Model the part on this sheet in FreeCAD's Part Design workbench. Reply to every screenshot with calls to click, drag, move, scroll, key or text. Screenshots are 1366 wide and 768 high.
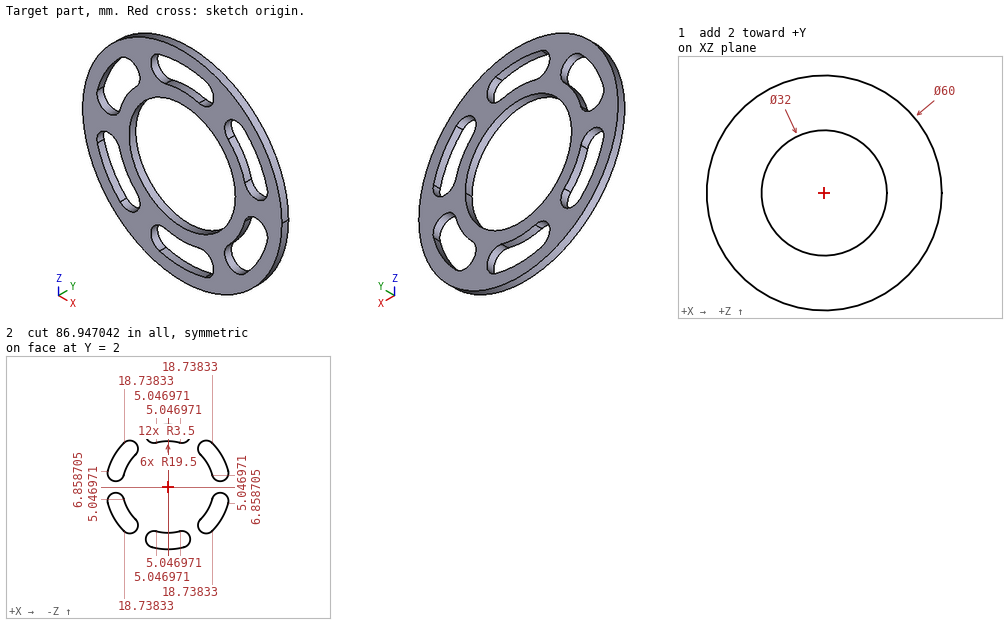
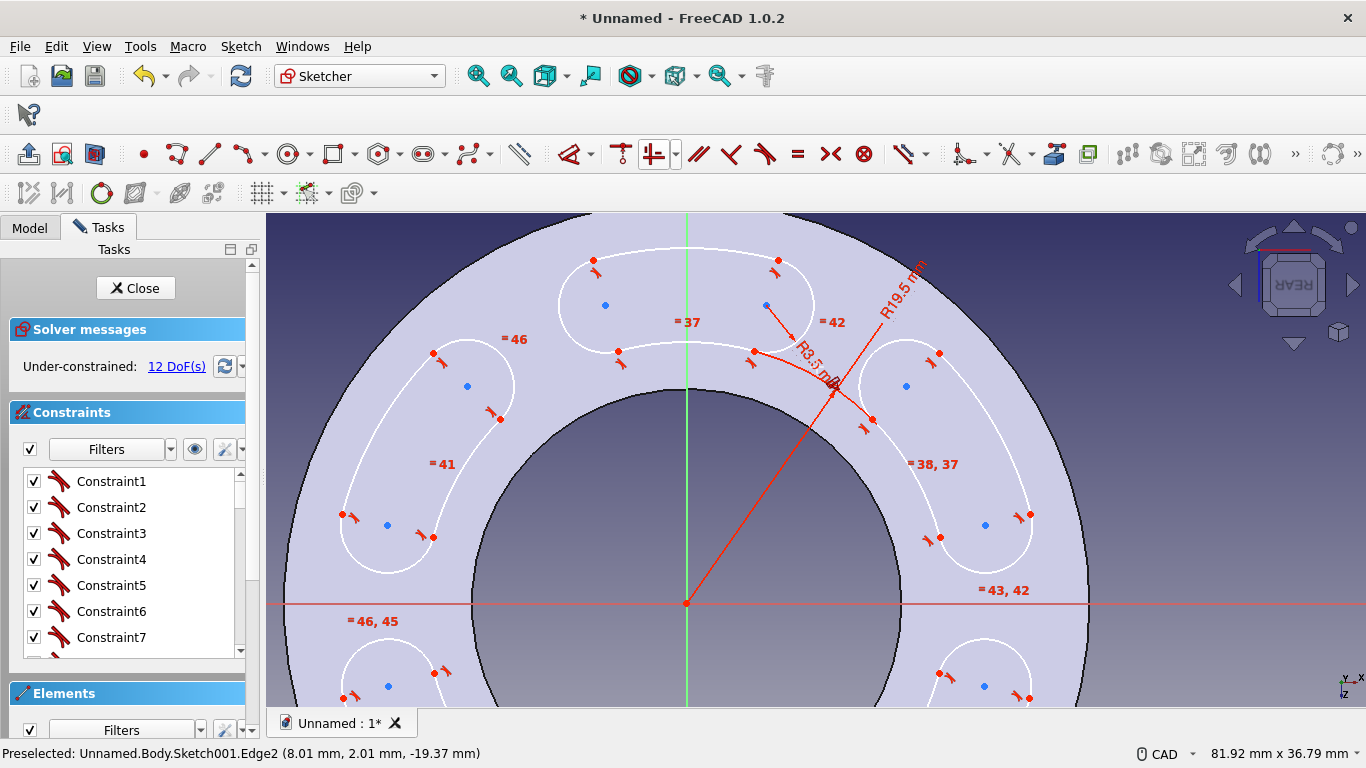
click(755, 351)
click(721, 317)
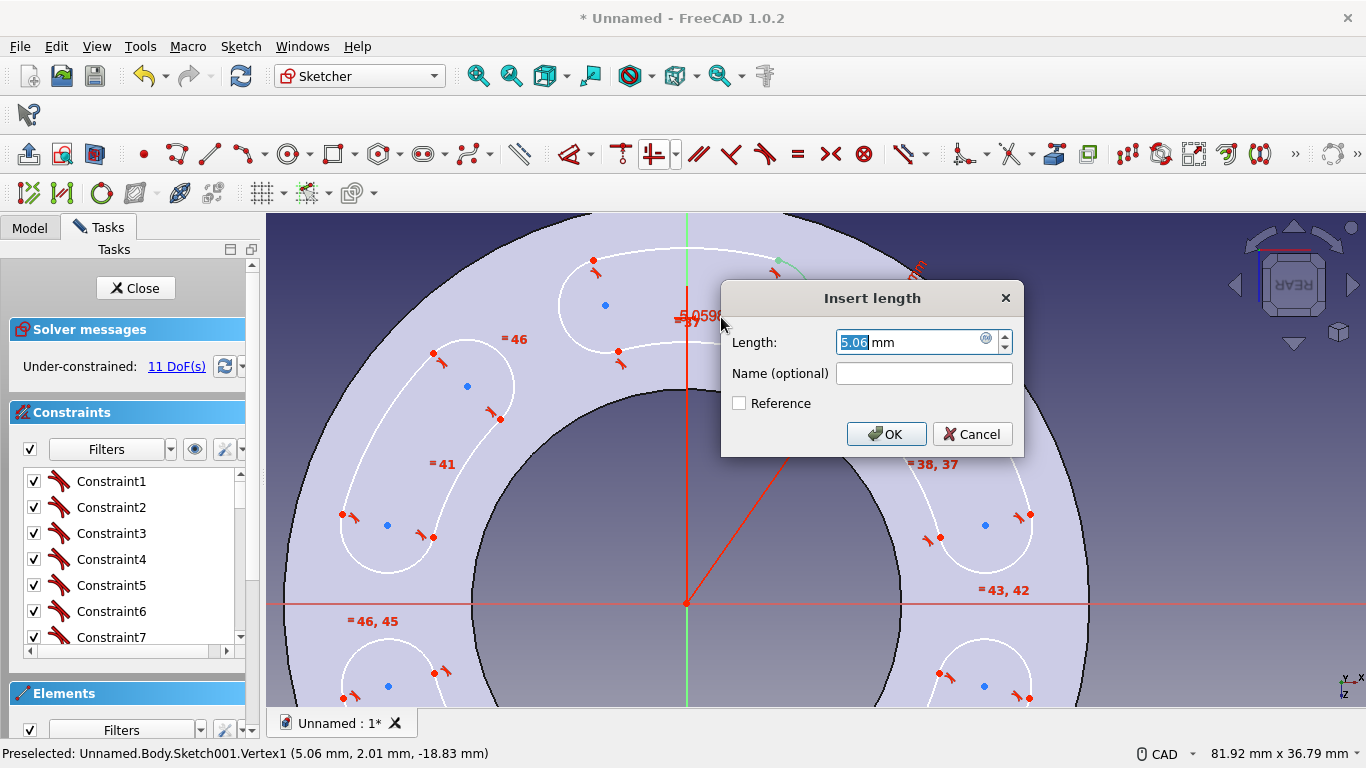
text(5.046971)
key(Return)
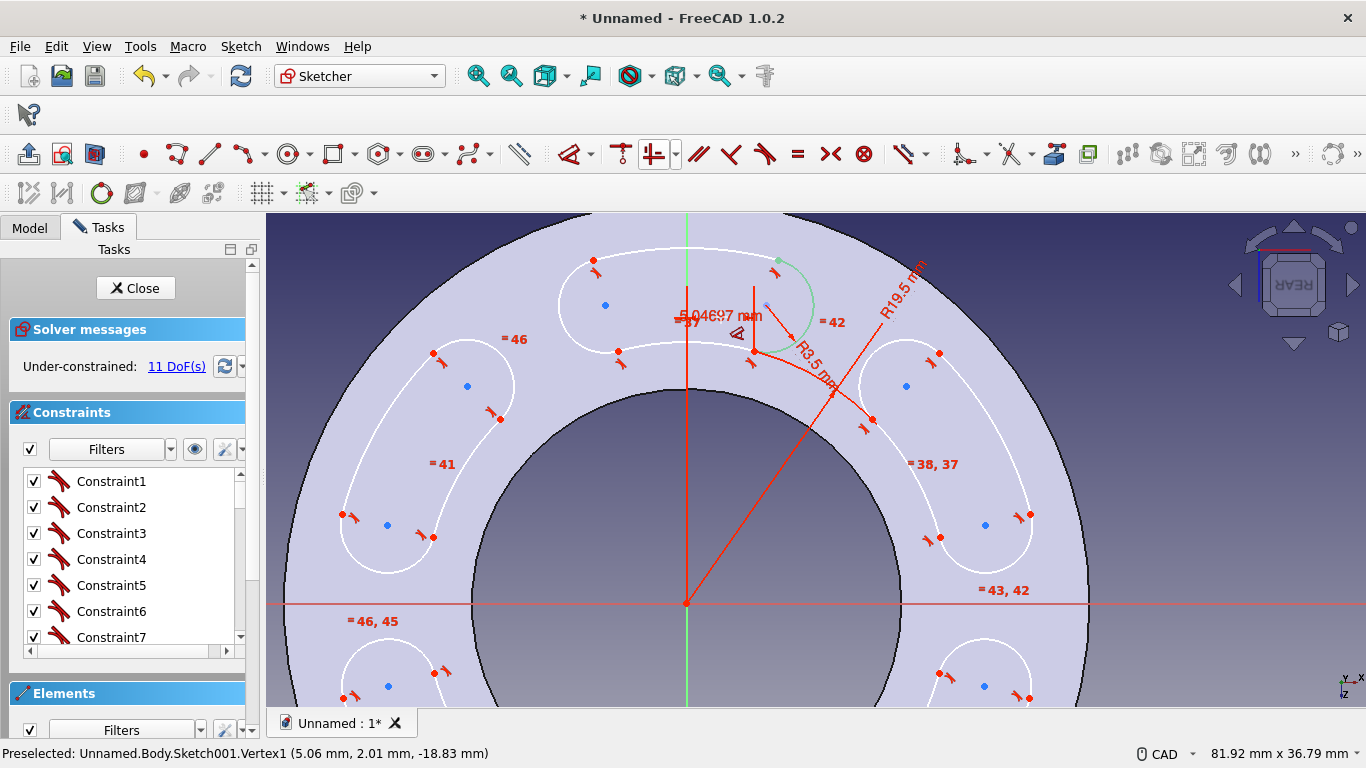
click(618, 351)
click(637, 317)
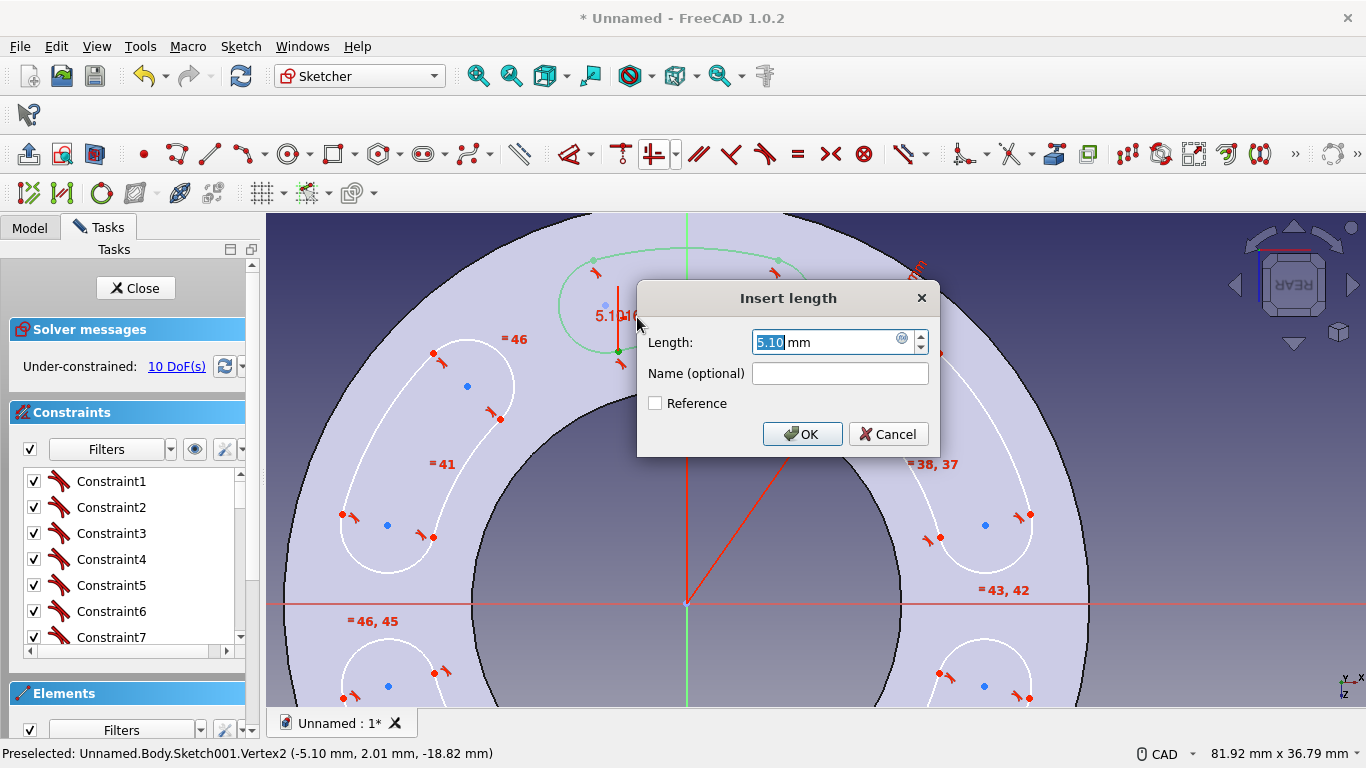
text(5.046971)
key(Return)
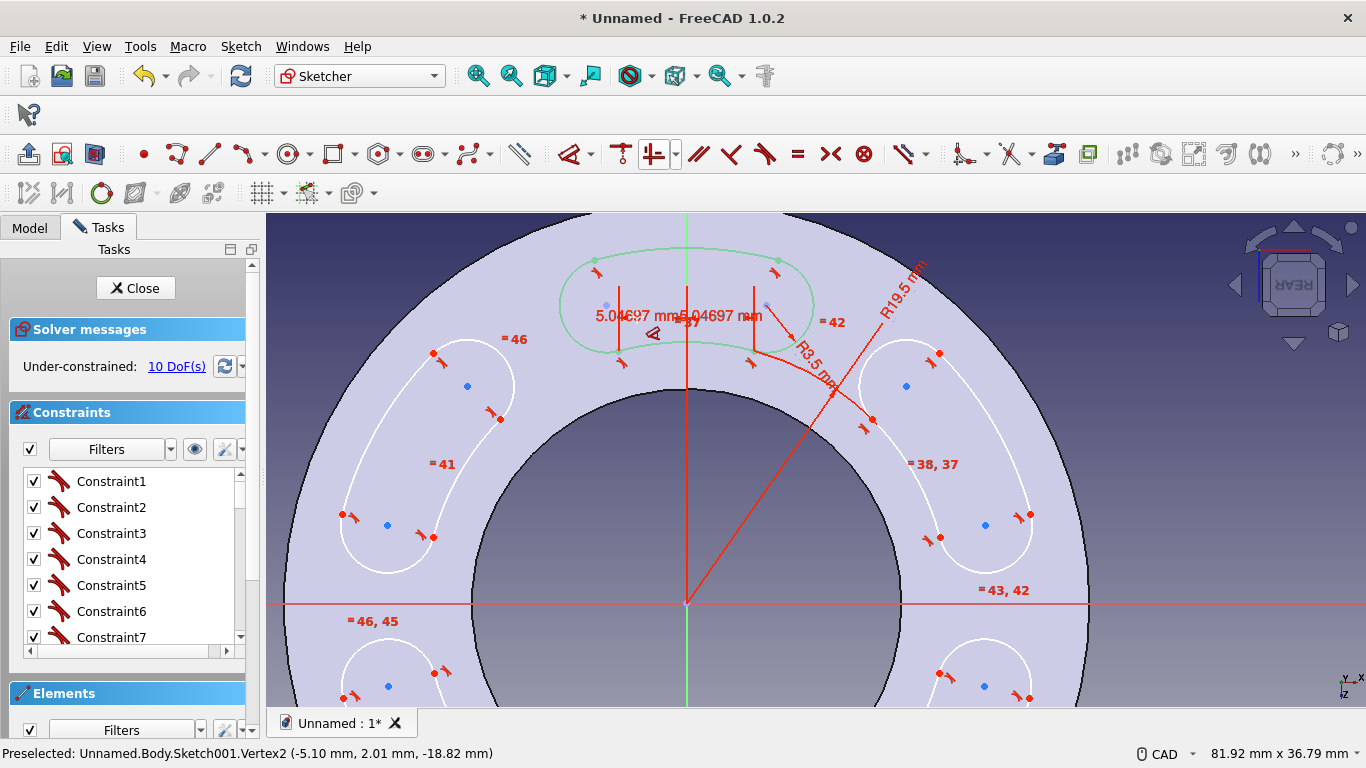
click(940, 538)
click(974, 556)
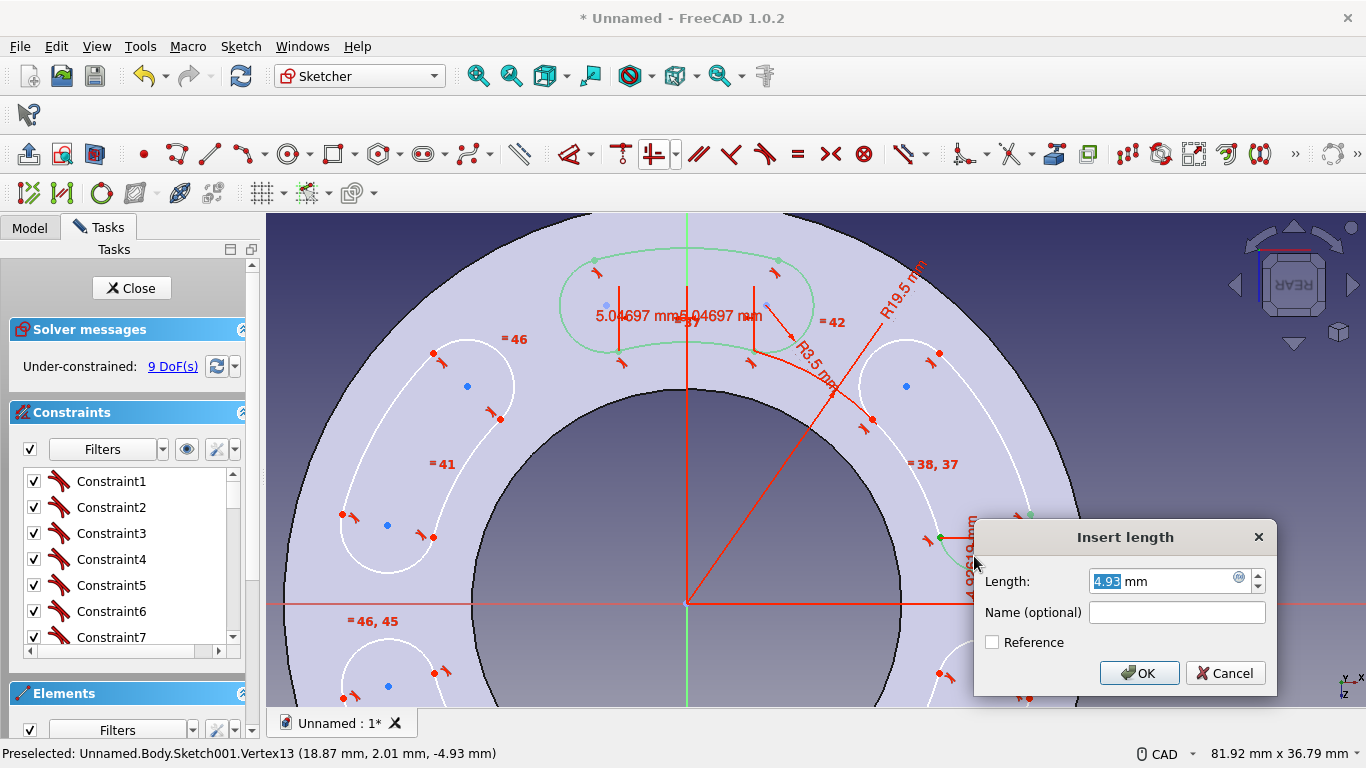
text(5.046971)
key(Return)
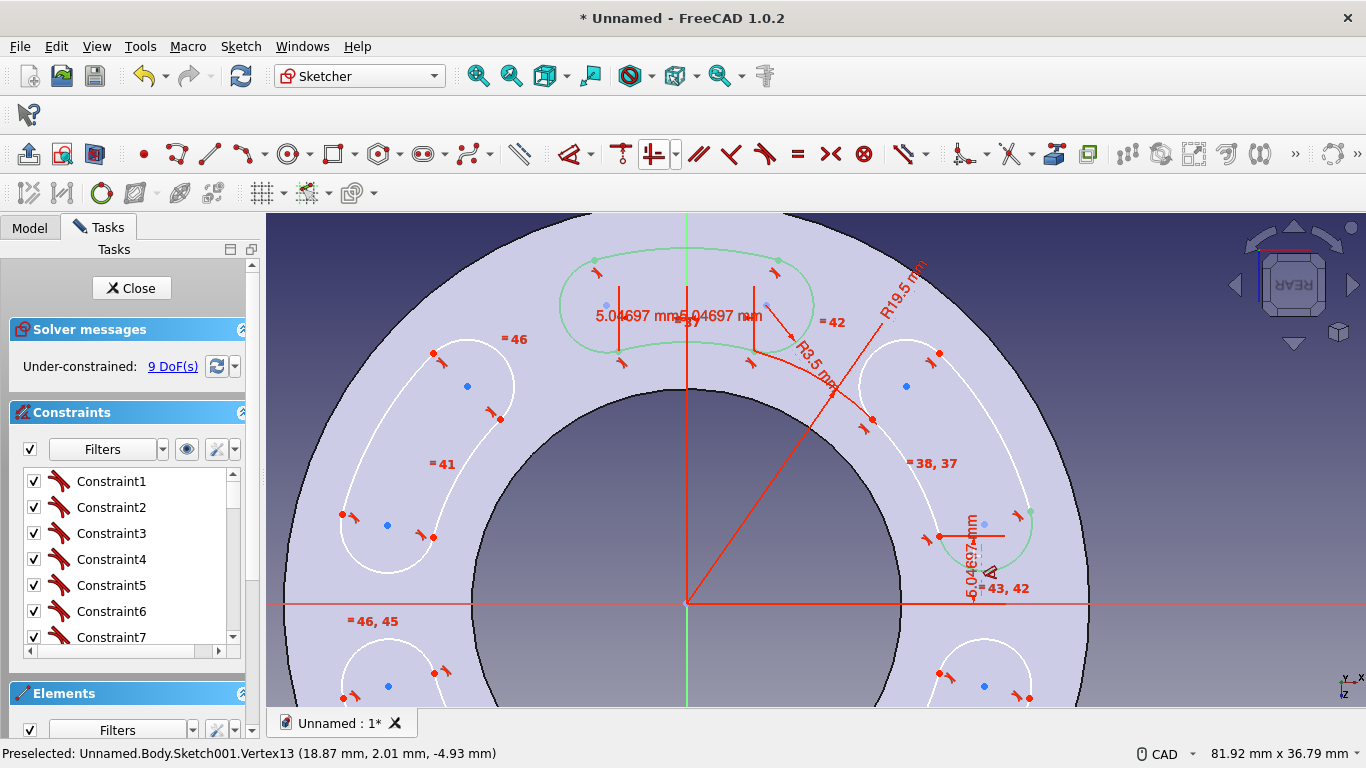
click(940, 354)
click(871, 320)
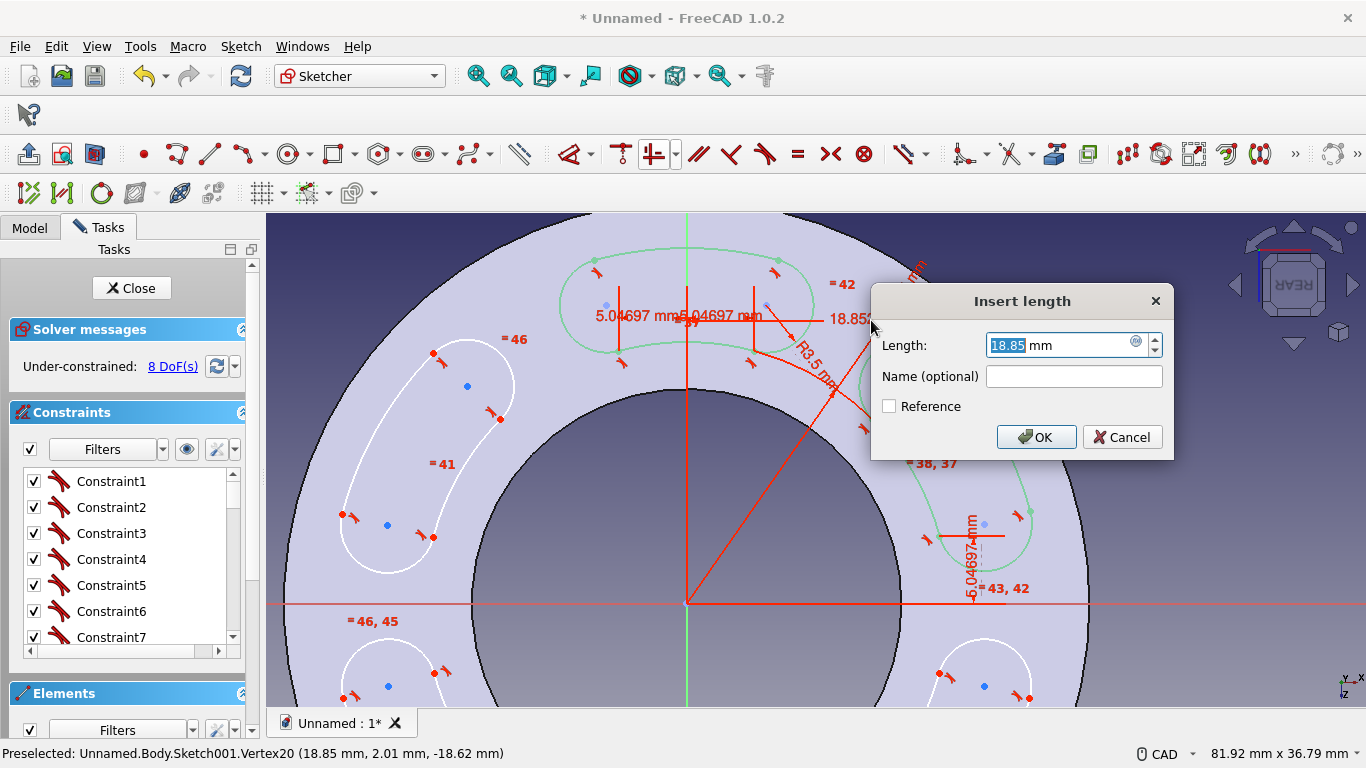
text(18.73833)
key(Return)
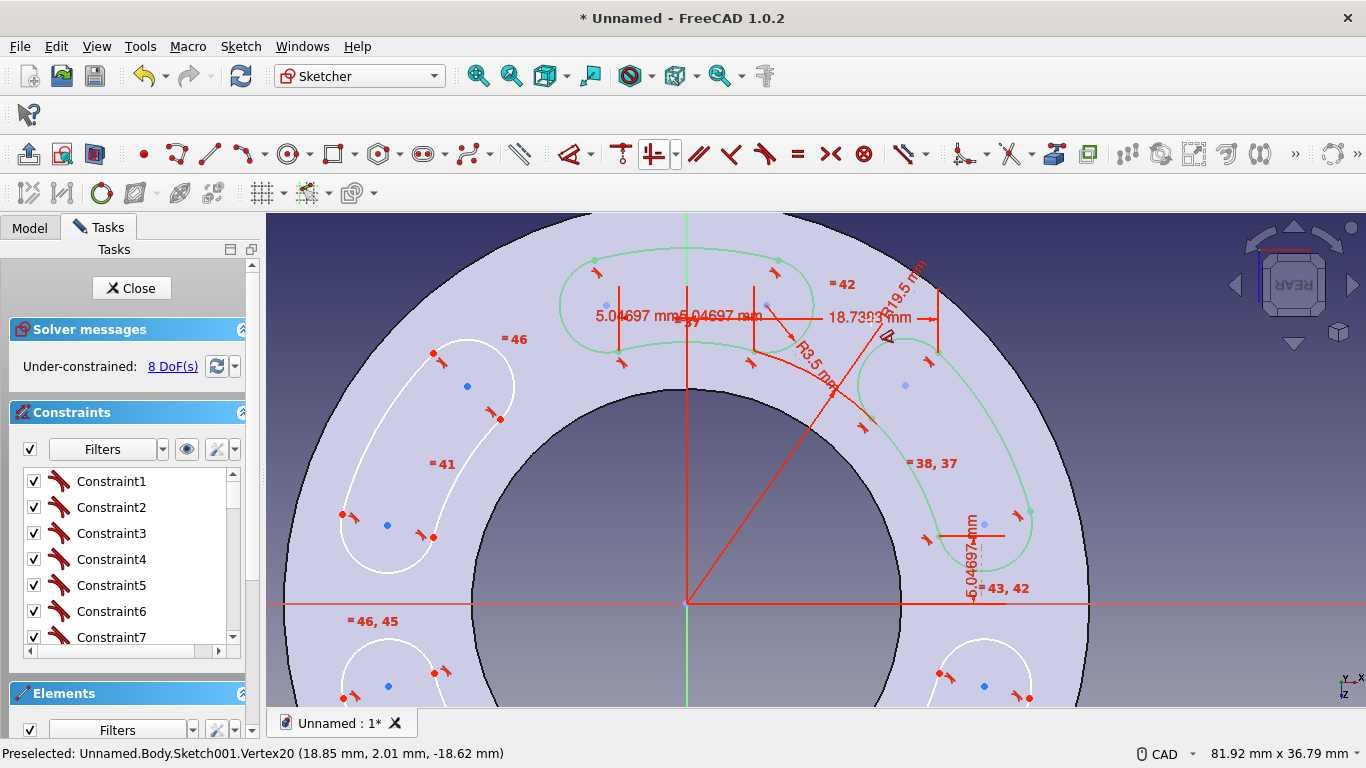
scroll(797, 343, down, 4)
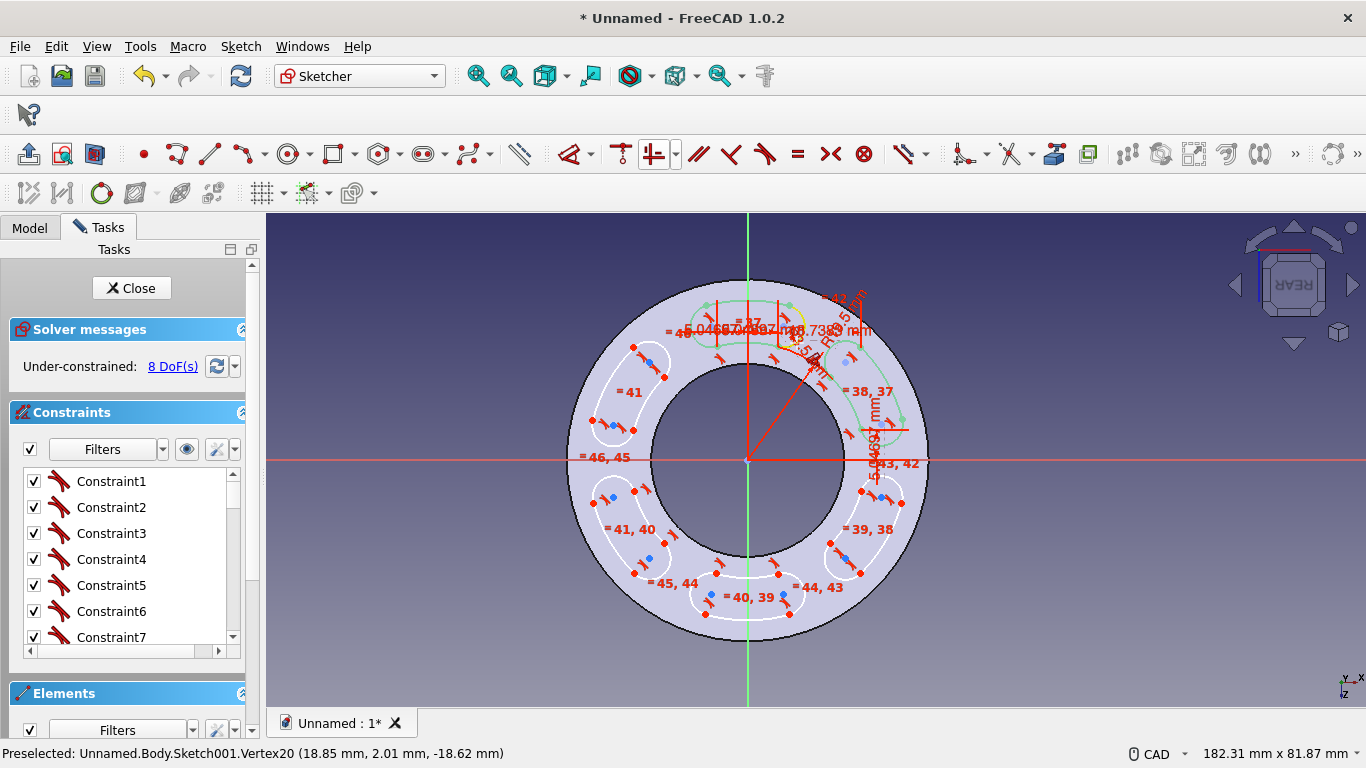
click(861, 574)
click(830, 608)